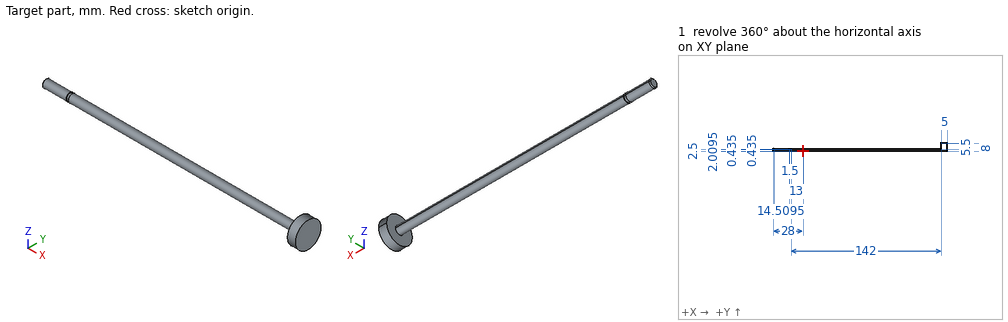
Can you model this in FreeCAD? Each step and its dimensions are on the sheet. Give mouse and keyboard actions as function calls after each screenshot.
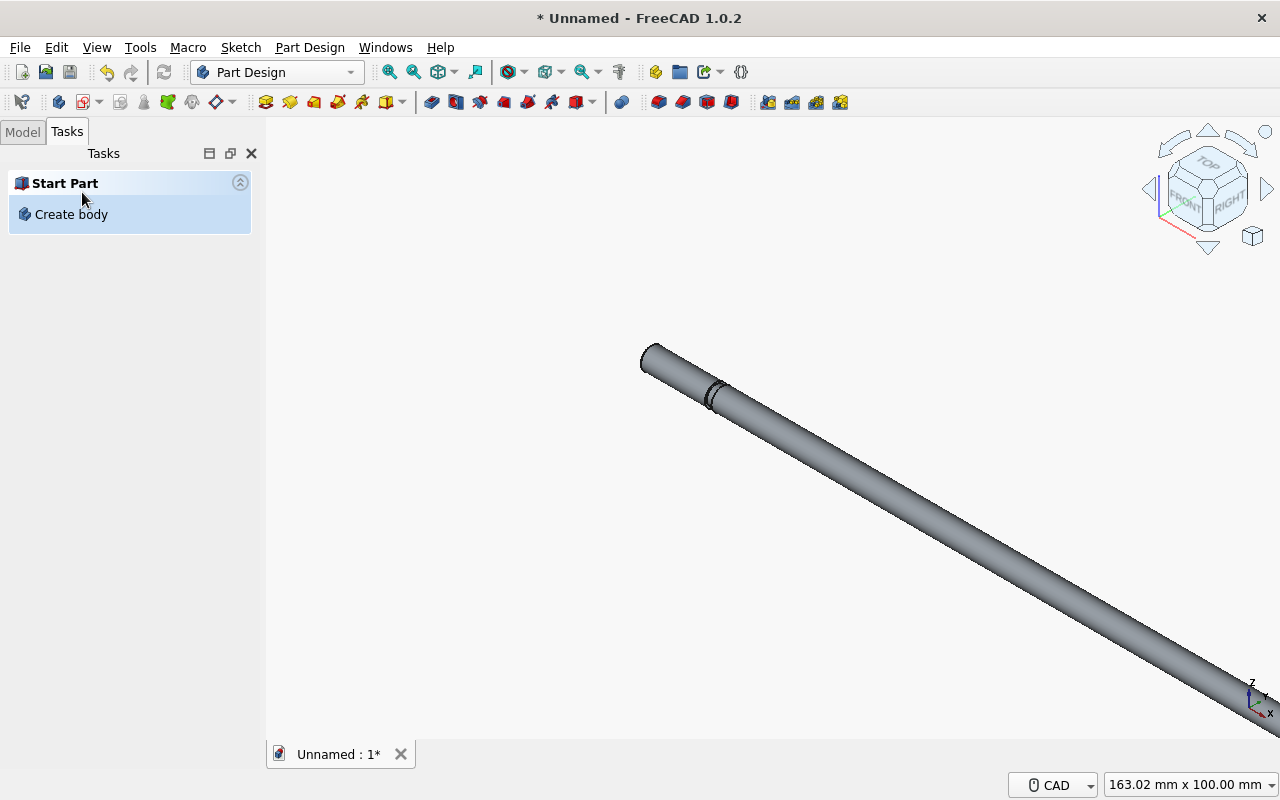
key(v)
key(f)